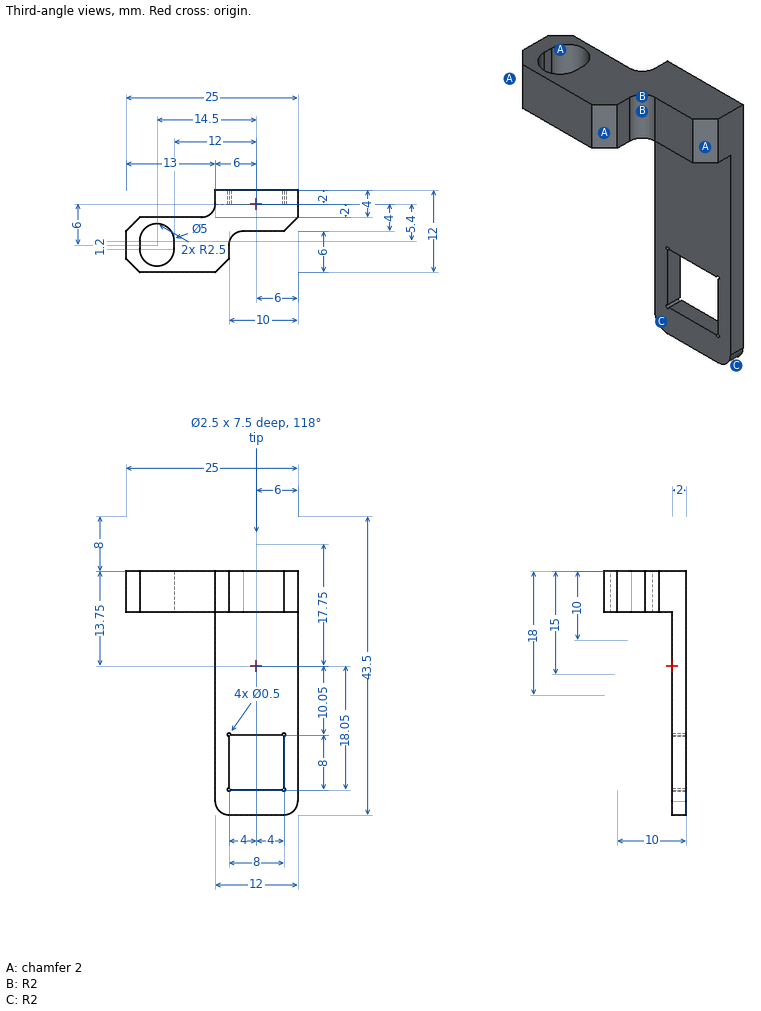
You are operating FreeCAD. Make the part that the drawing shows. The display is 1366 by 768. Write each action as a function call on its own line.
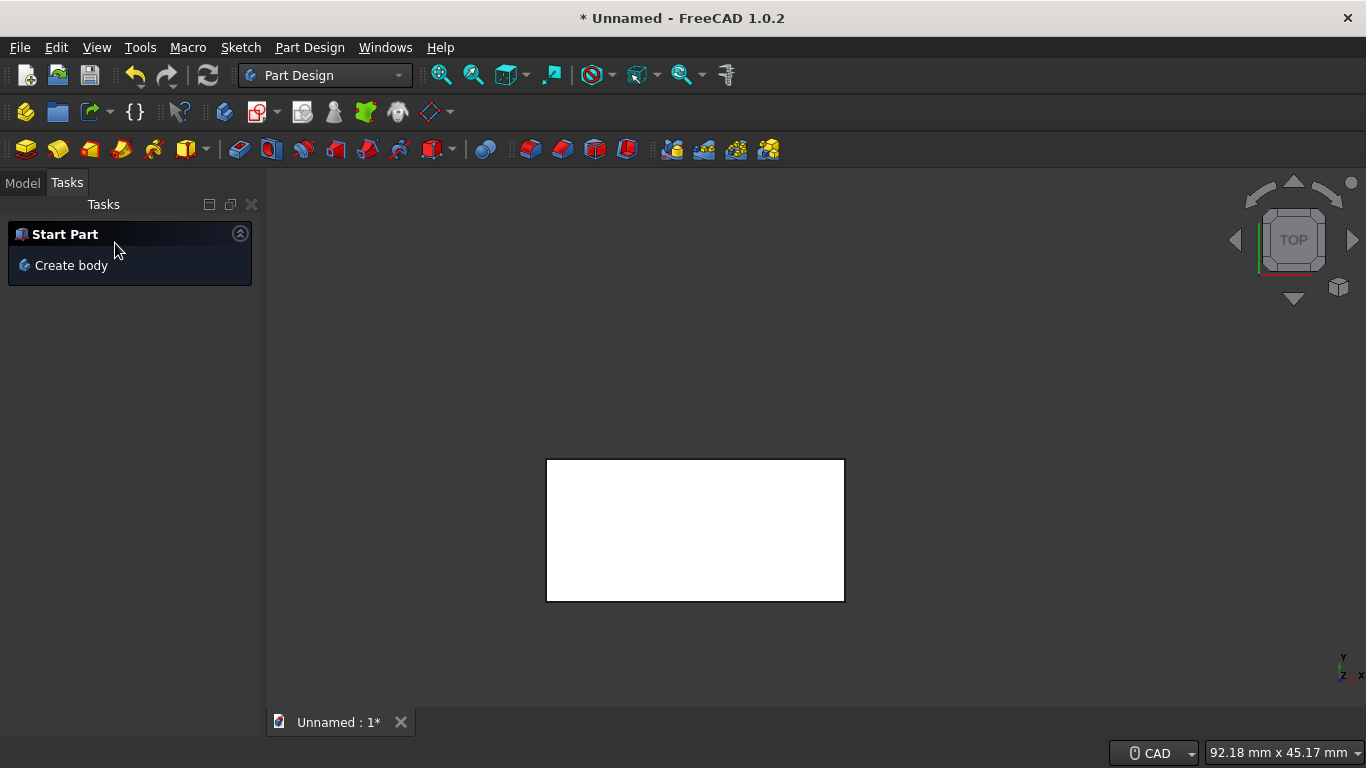
click(442, 76)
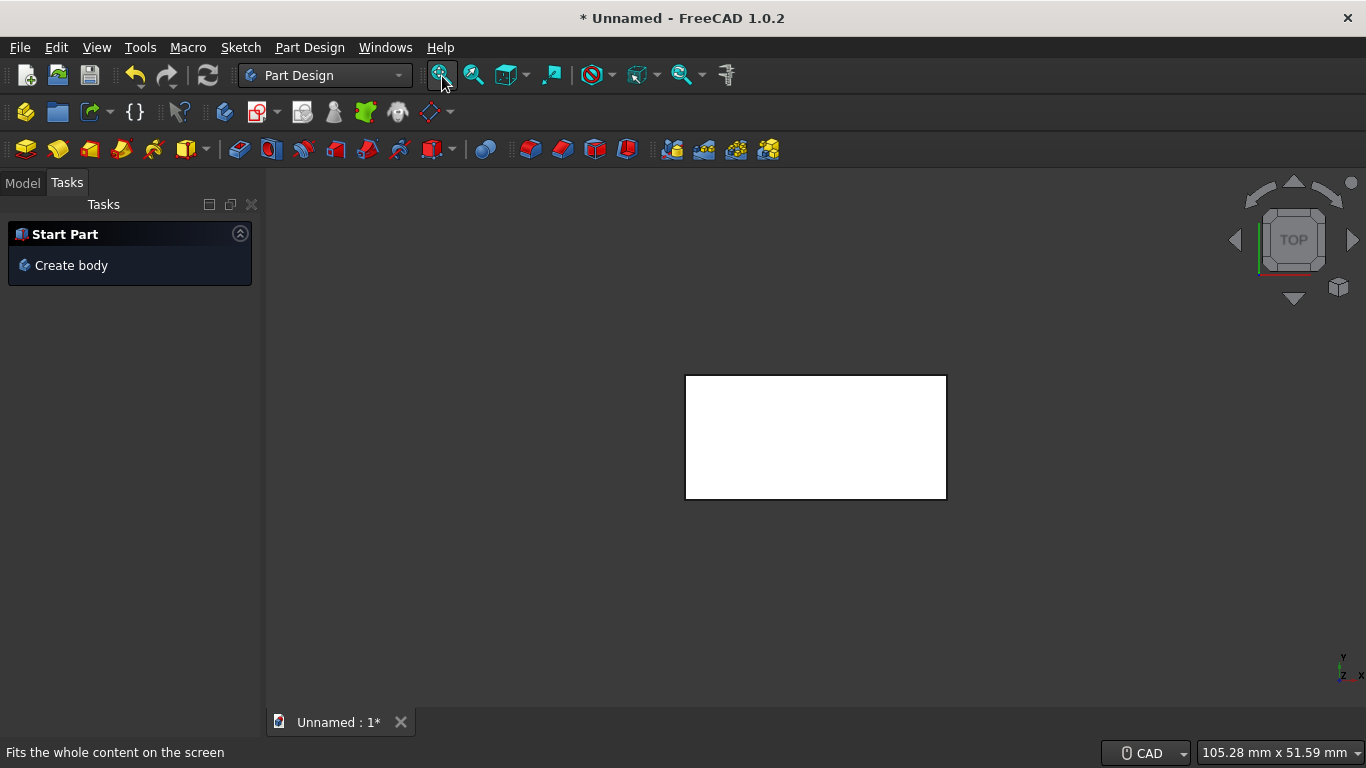
key(4)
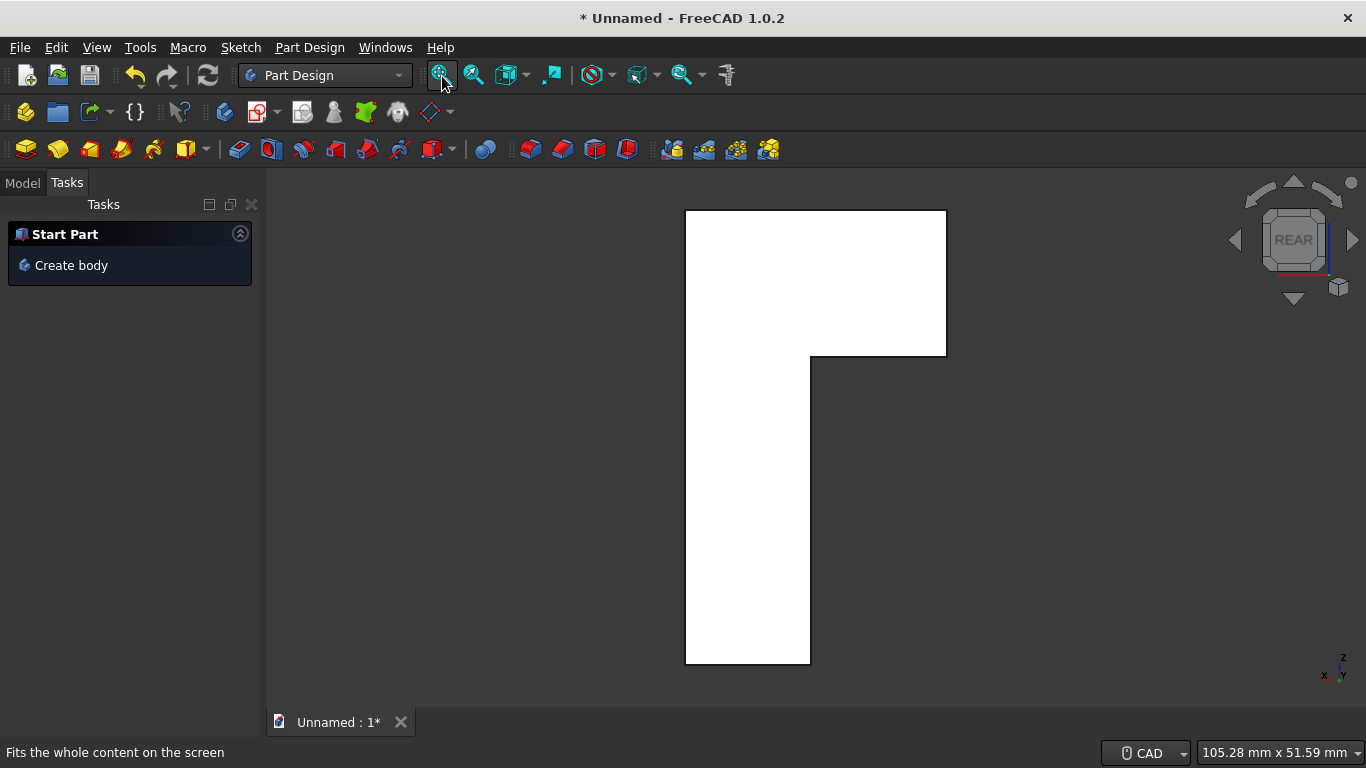
click(779, 307)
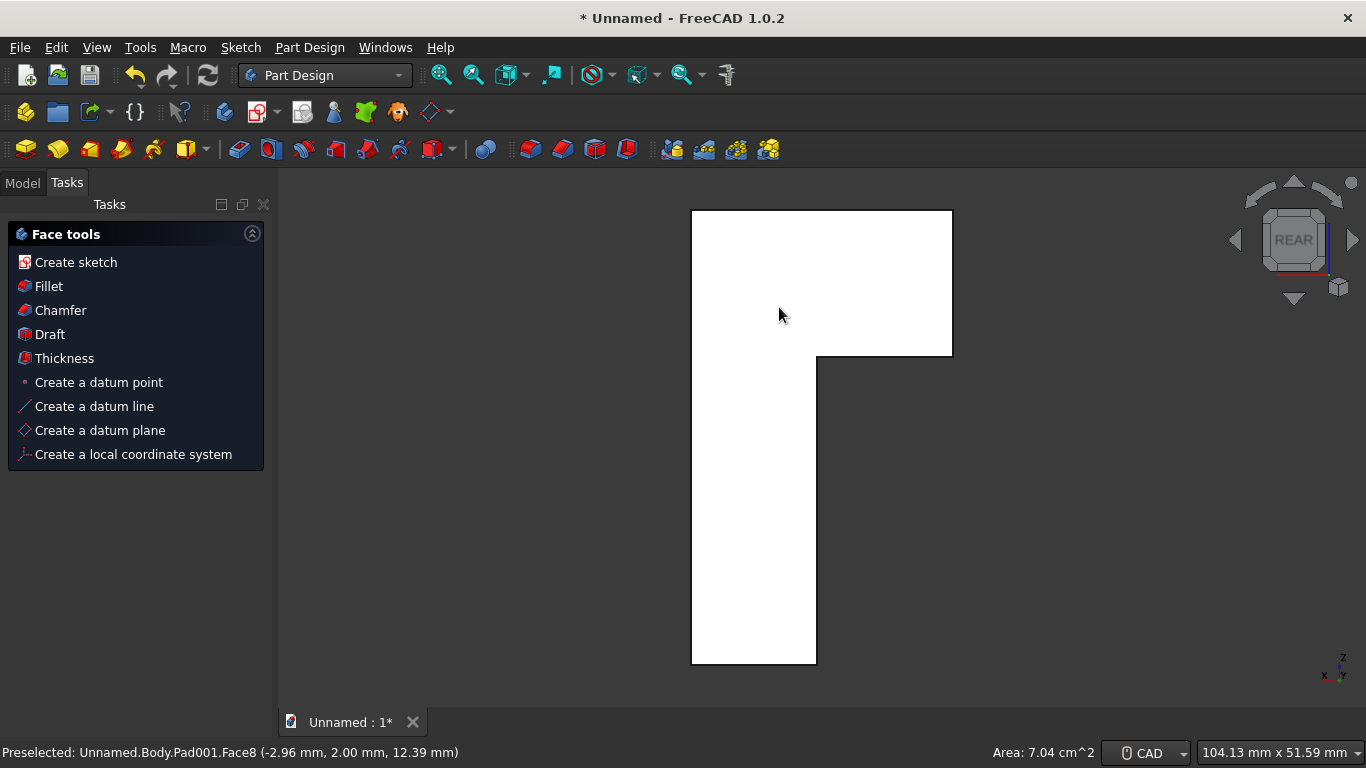
click(258, 112)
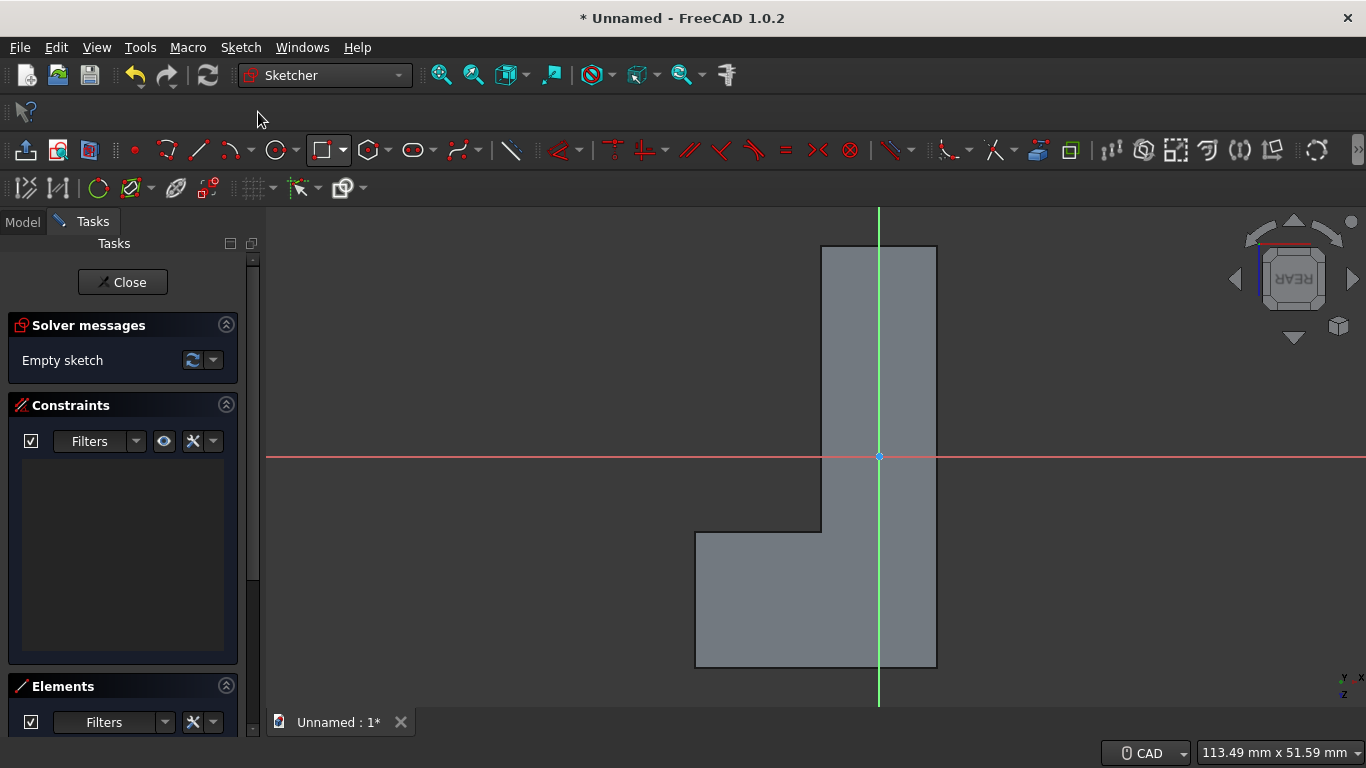
scroll(438, 235, down, 1)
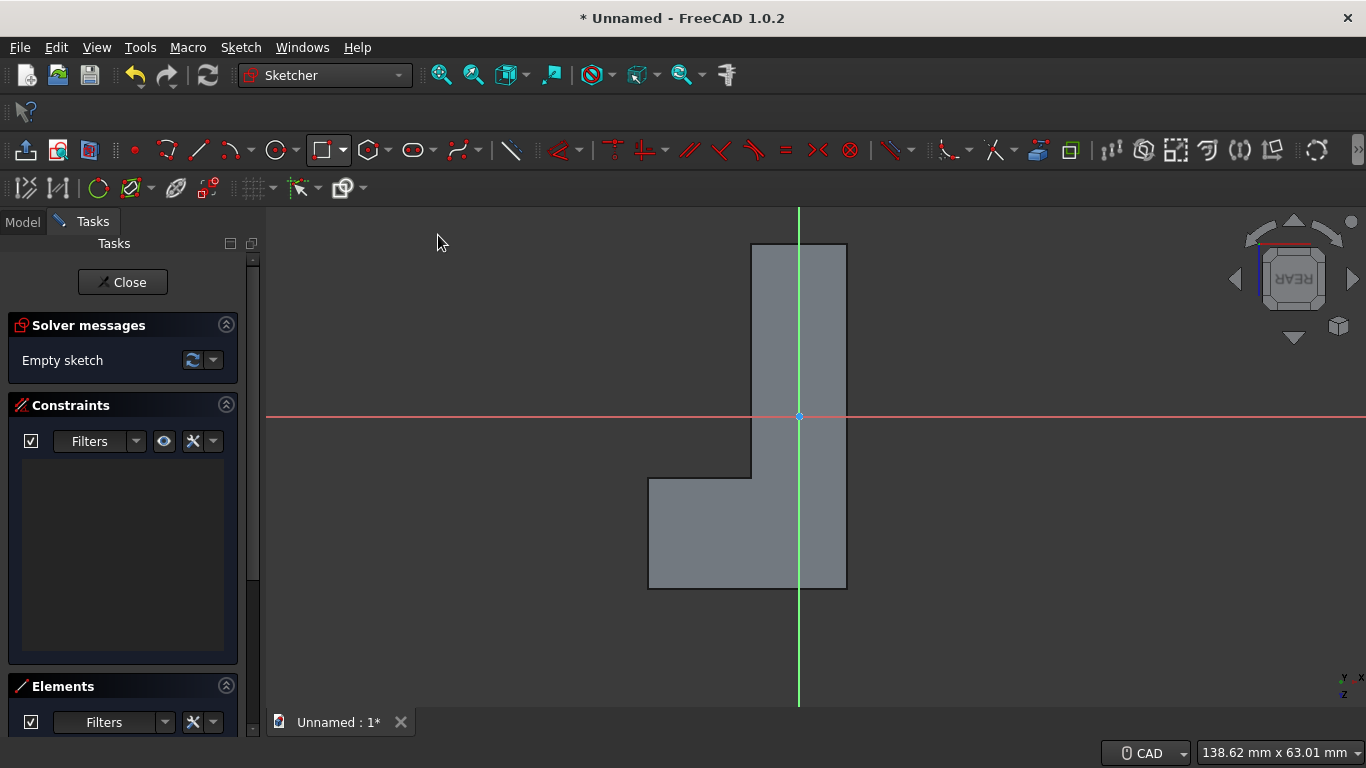
scroll(748, 559, up, 3)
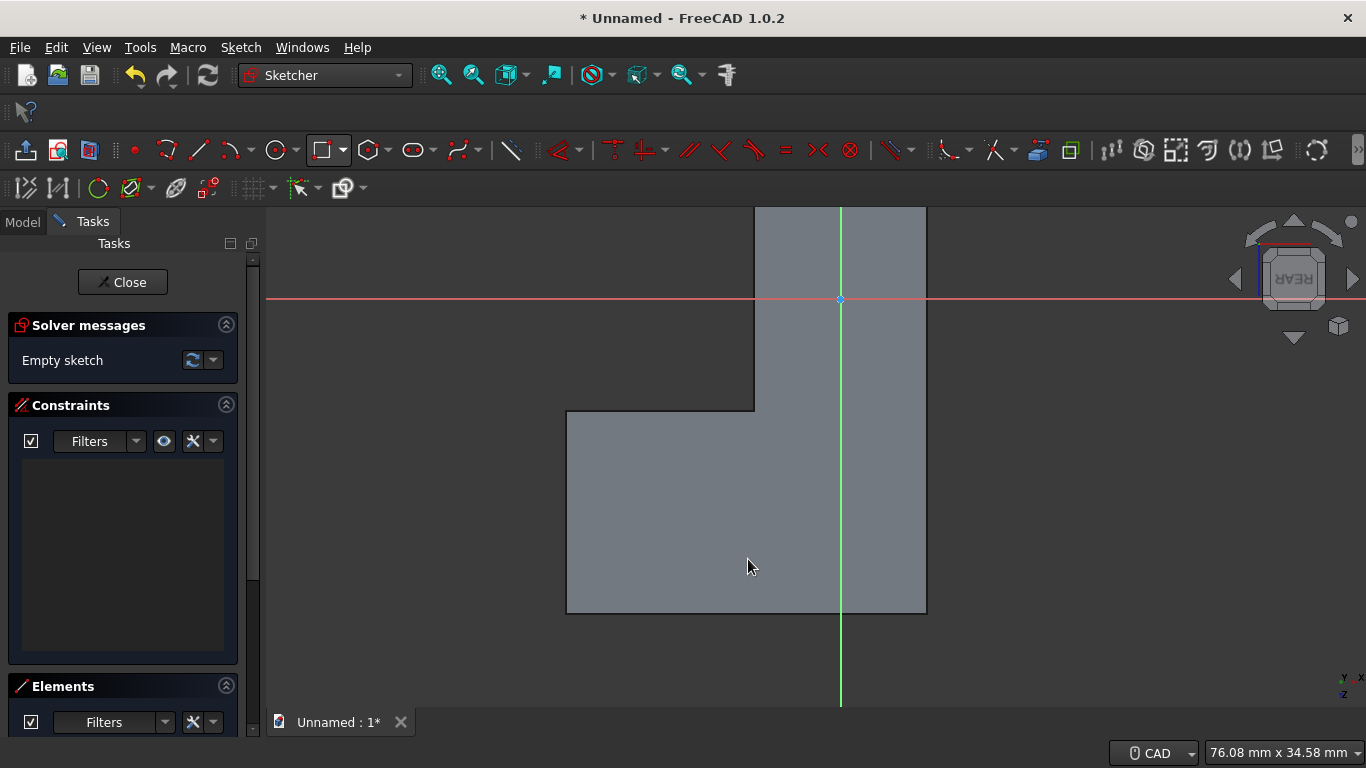
click(322, 150)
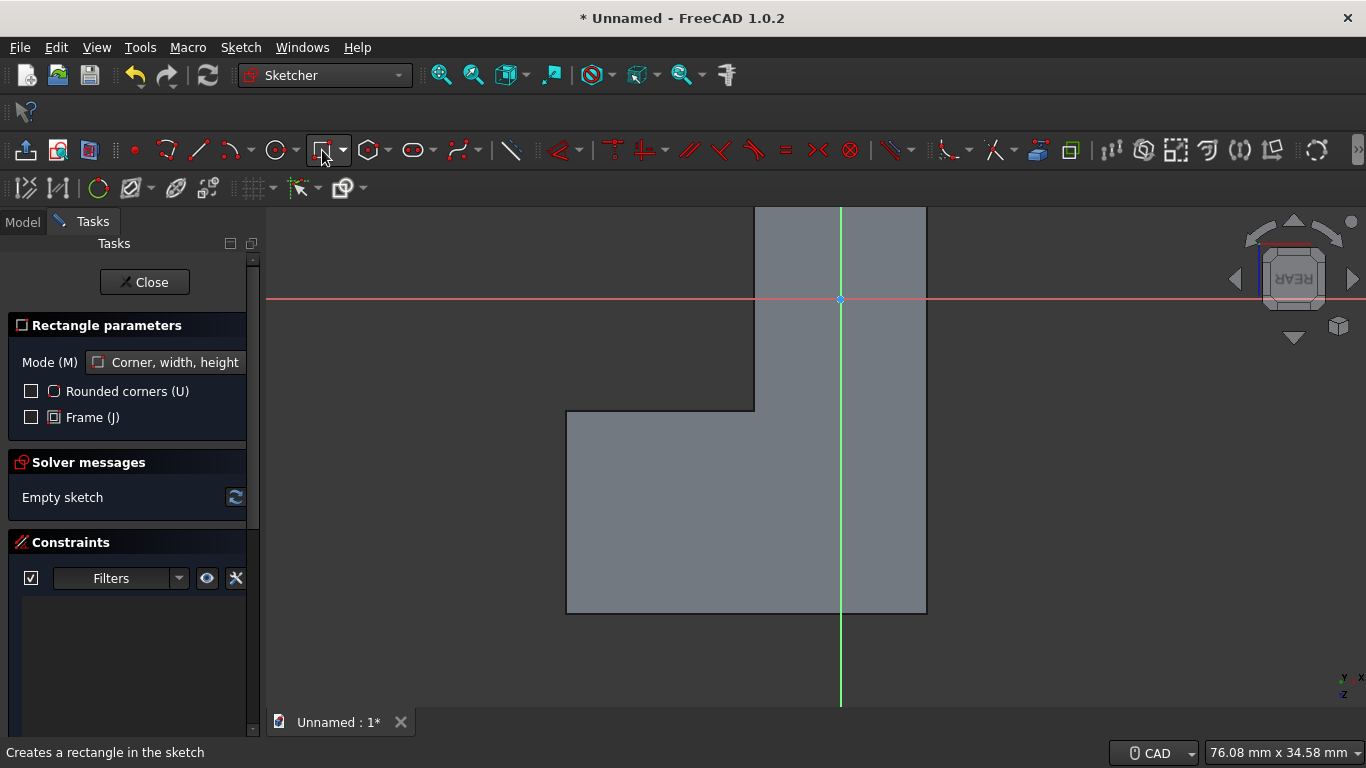
click(566, 498)
click(927, 614)
key(Escape)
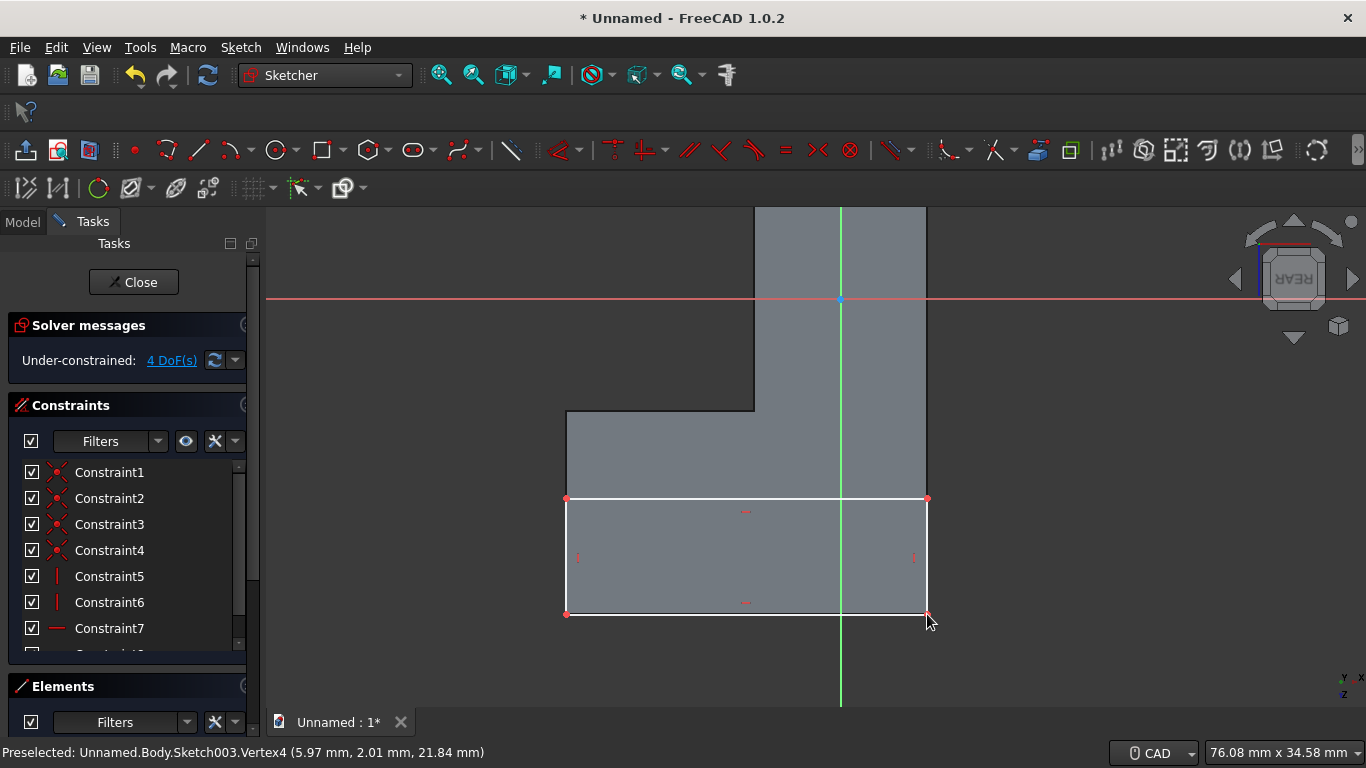
key(d)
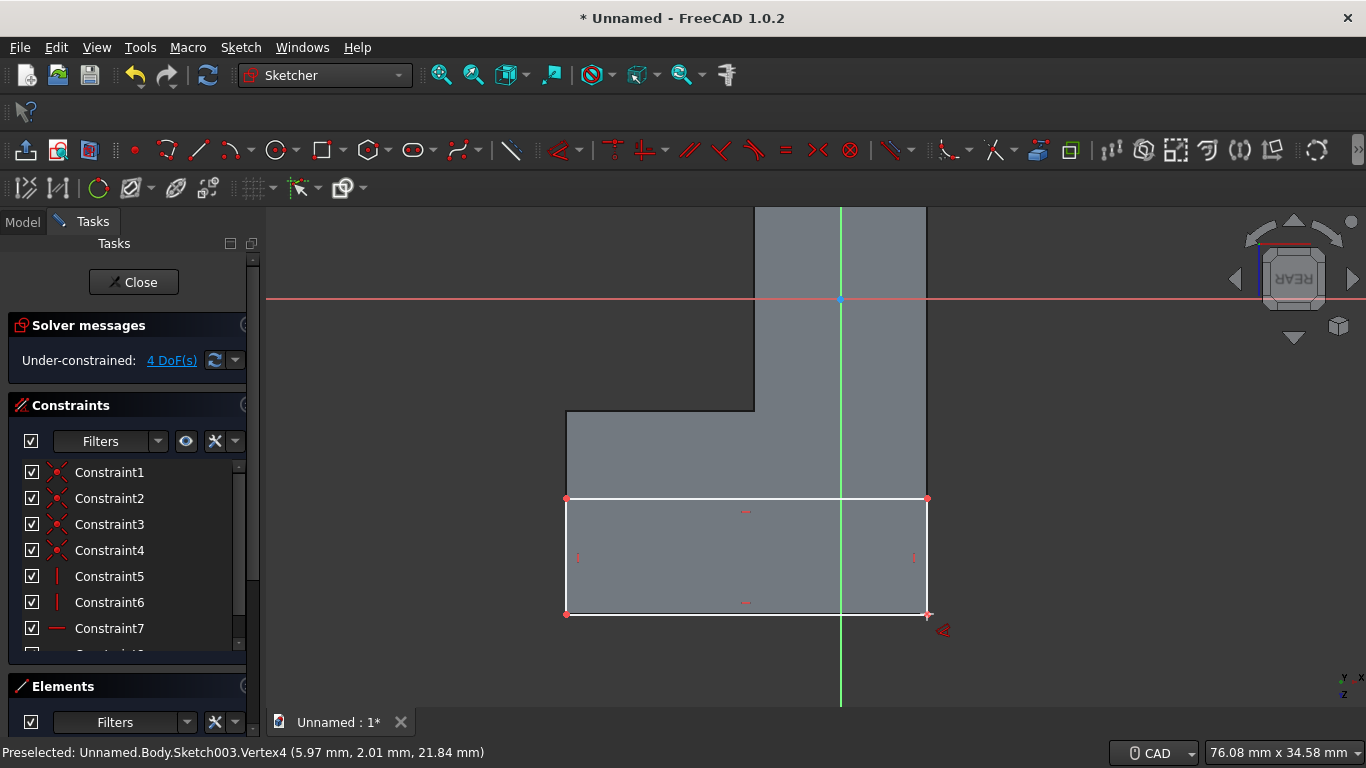
click(566, 534)
click(532, 557)